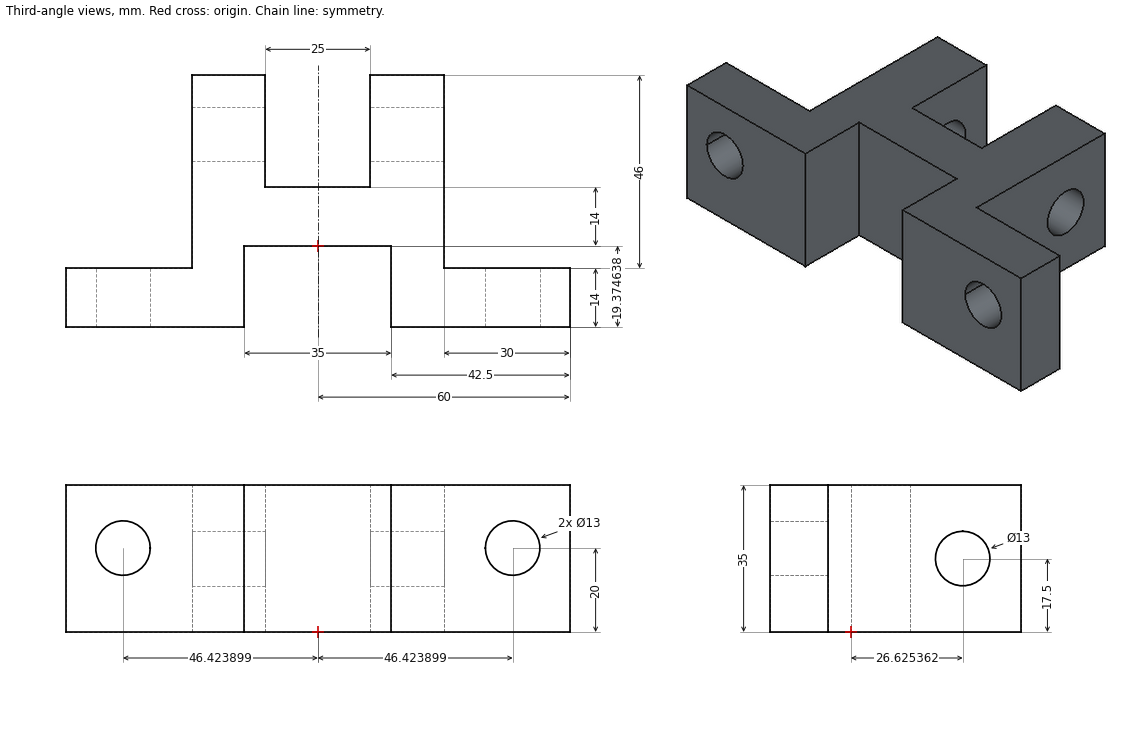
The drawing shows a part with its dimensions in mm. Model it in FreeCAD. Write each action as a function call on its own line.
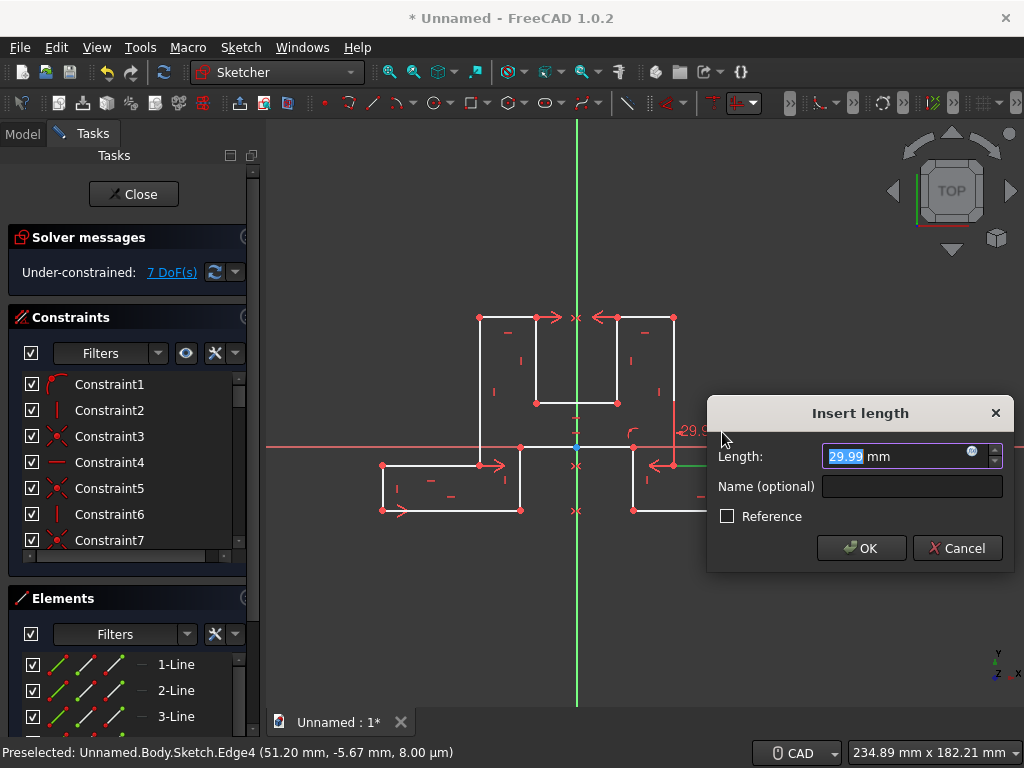
text(30)
key(Return)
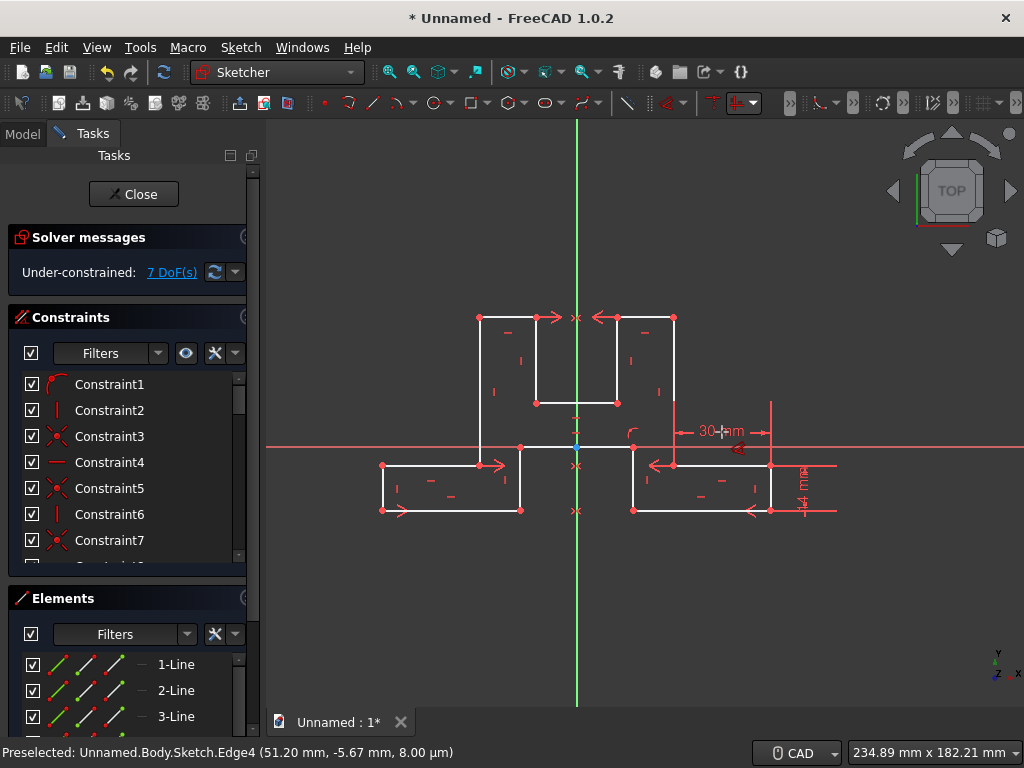
click(674, 421)
click(708, 392)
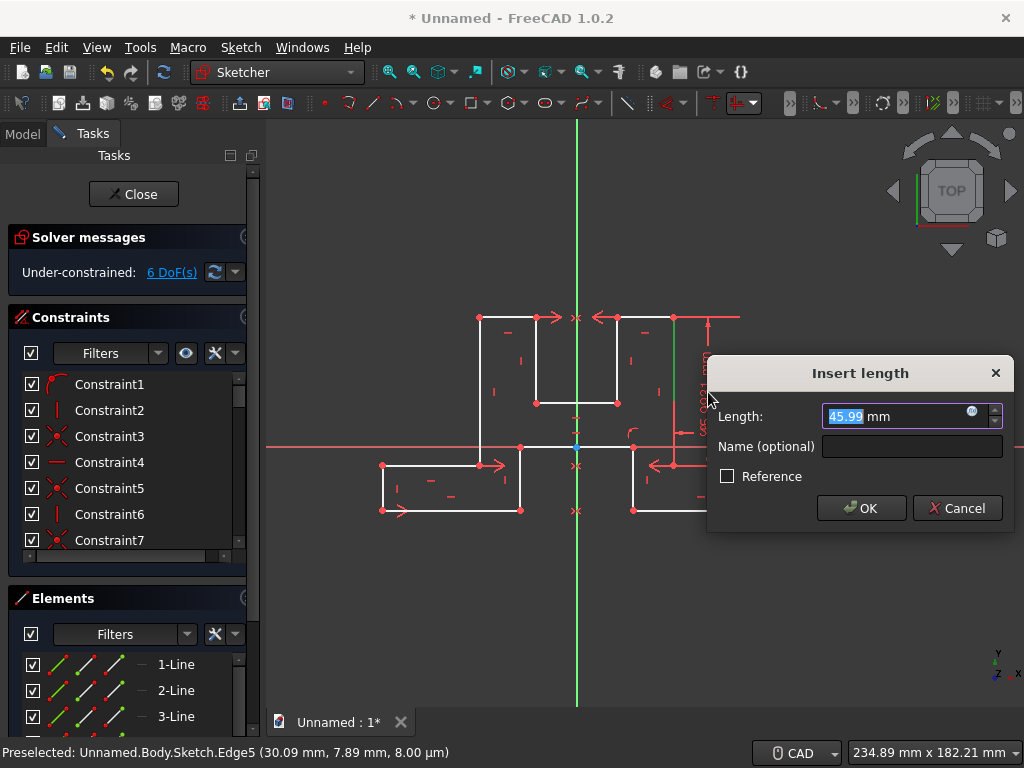
text(46)
key(Return)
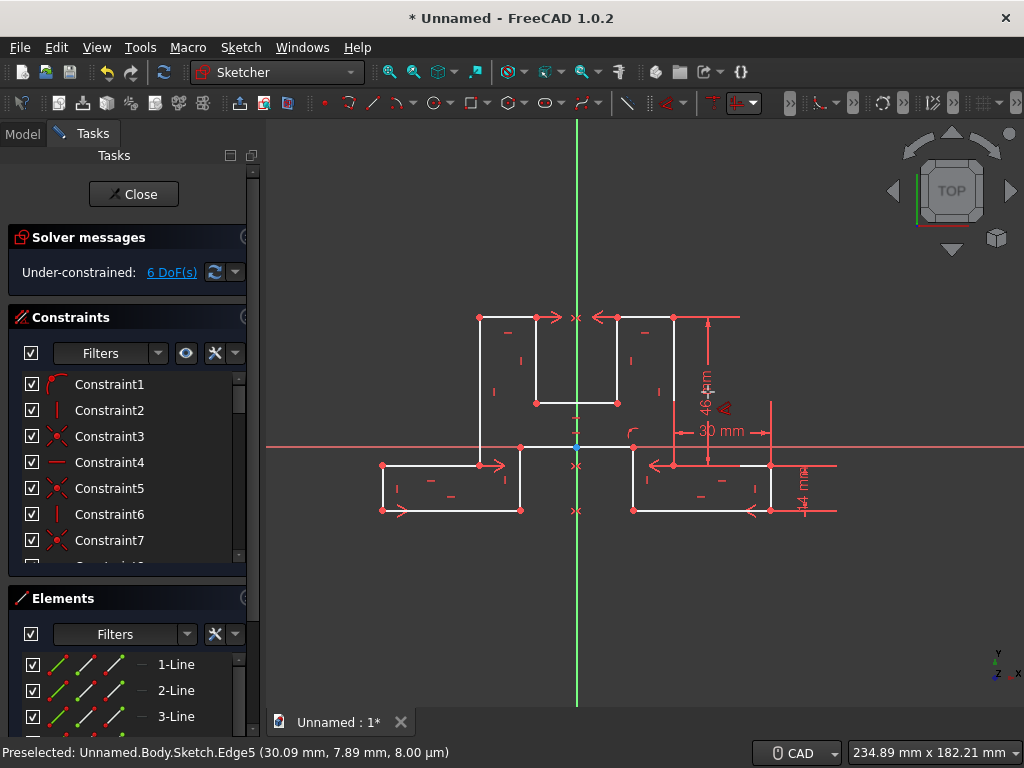
click(593, 403)
click(558, 369)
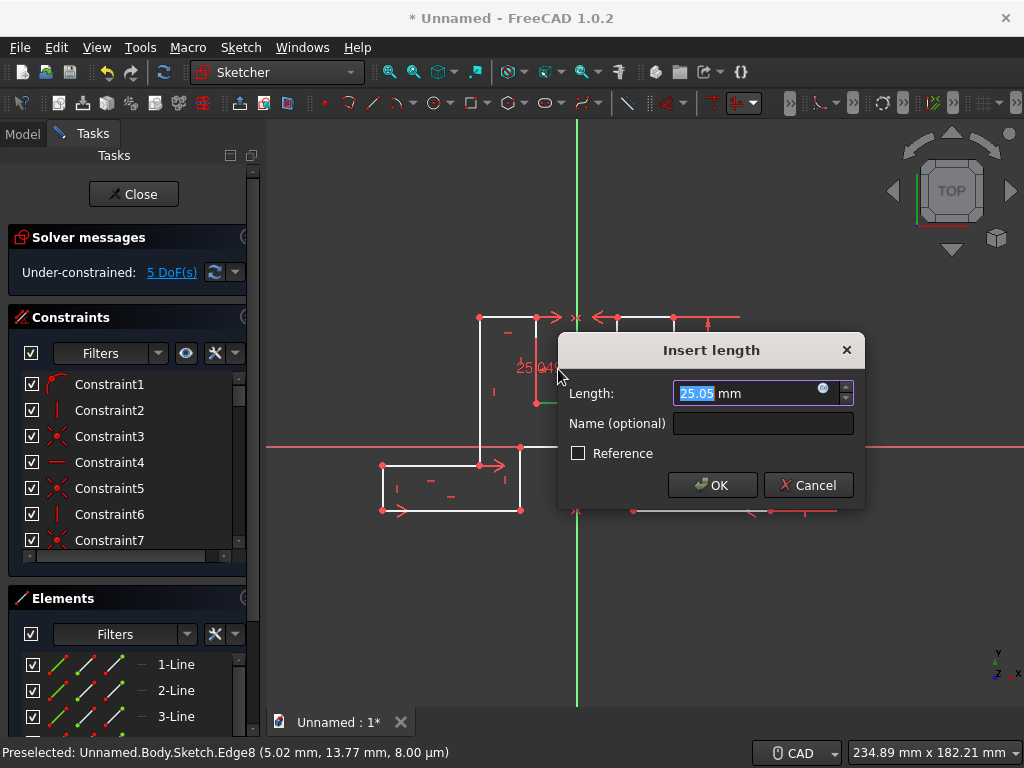
text(25)
key(Return)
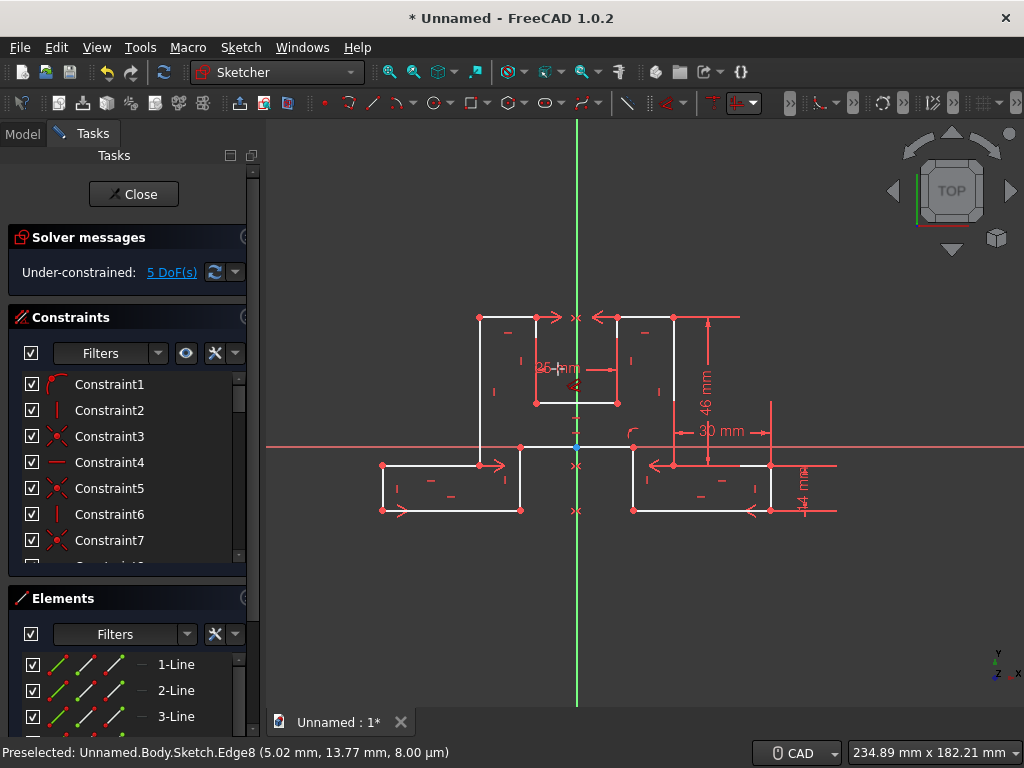
click(554, 447)
click(551, 481)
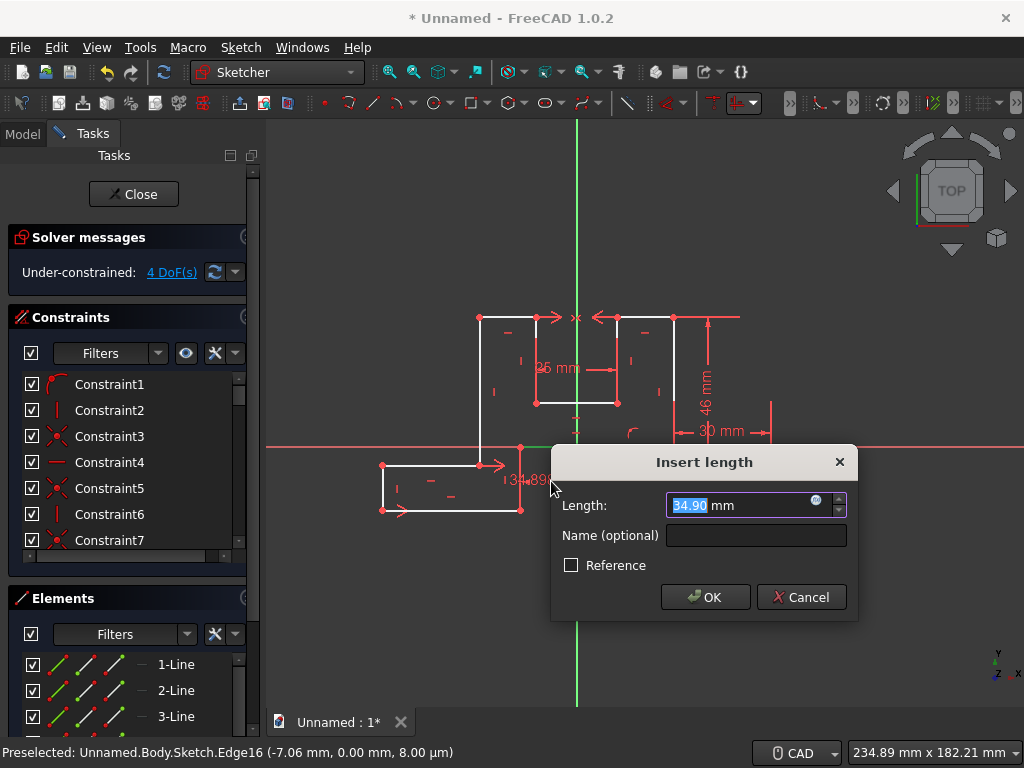
text(35)
key(Return)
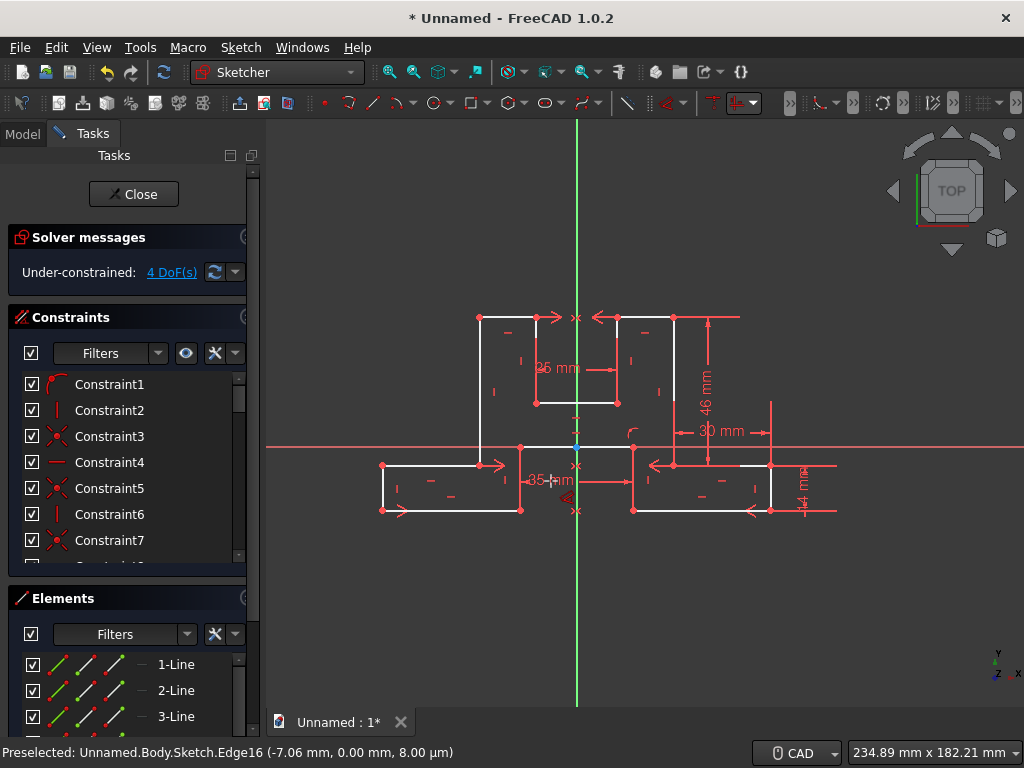
click(771, 511)
click(674, 545)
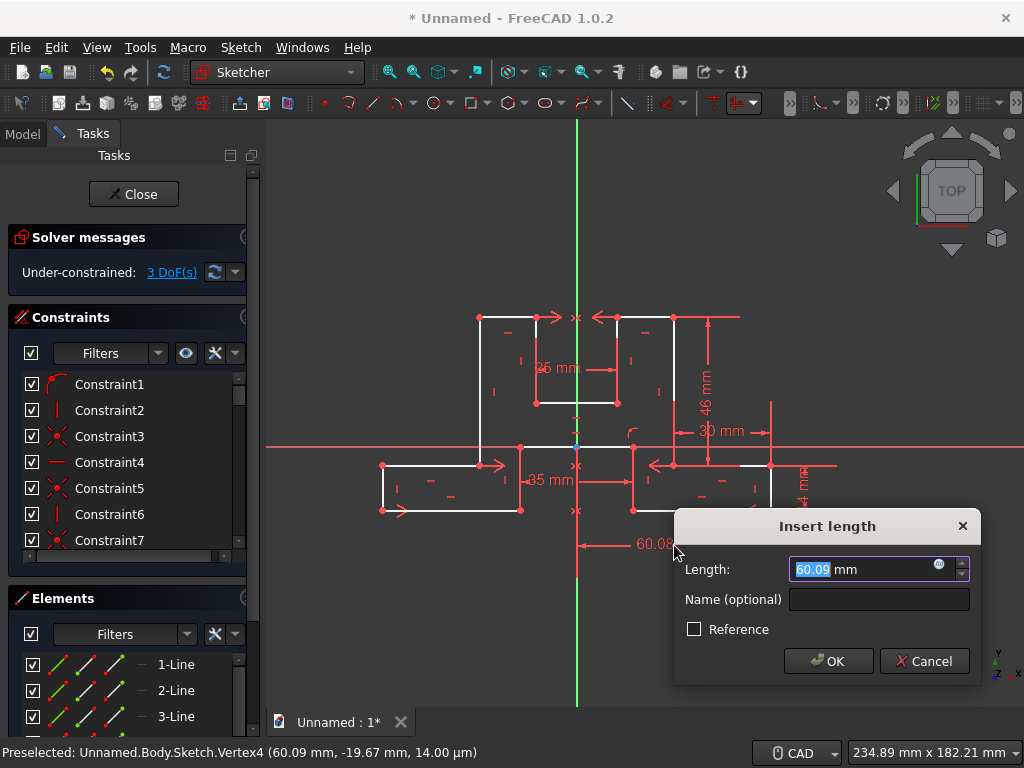
text(60)
key(Return)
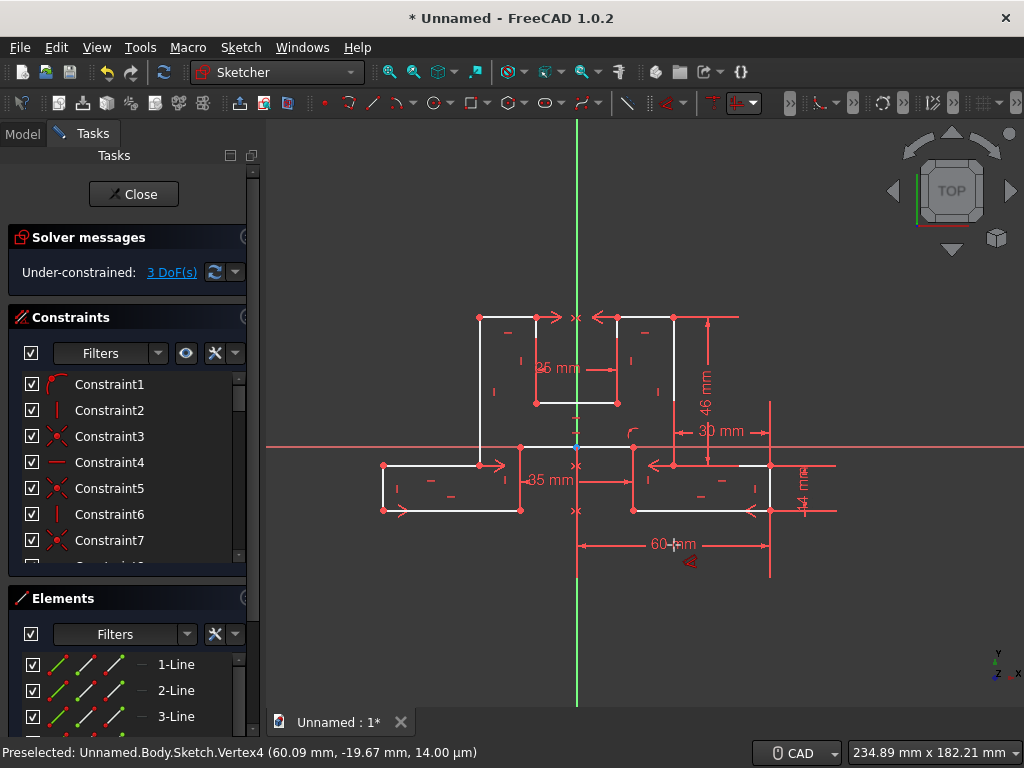
click(617, 403)
click(651, 425)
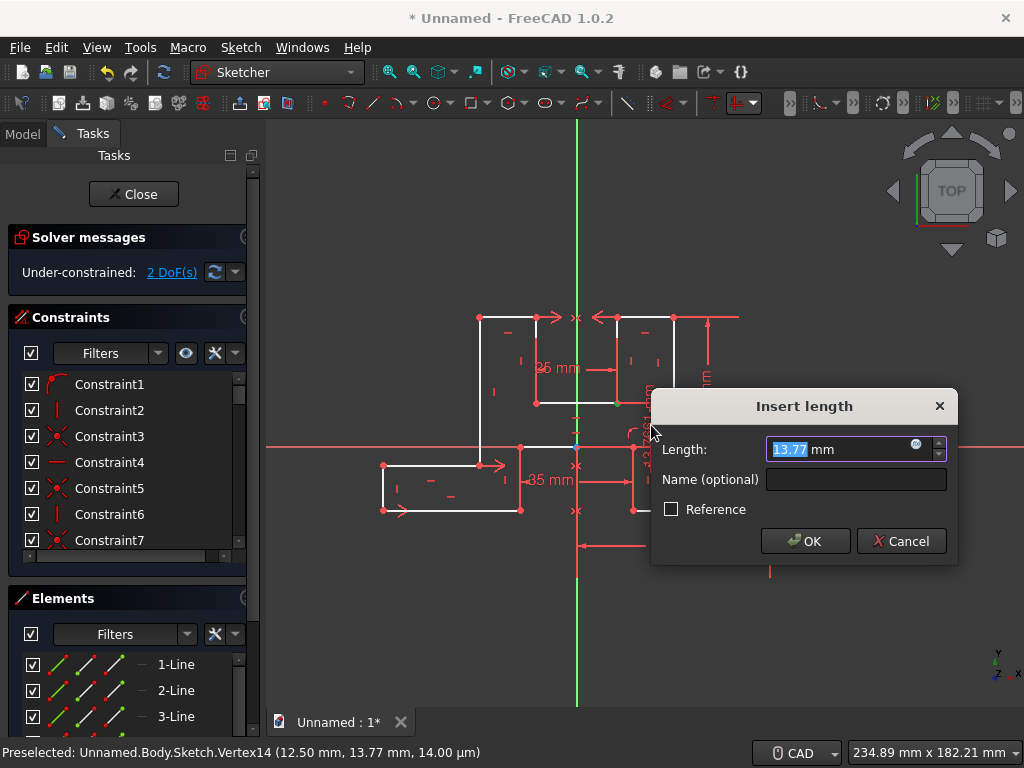
text(14)
key(Return)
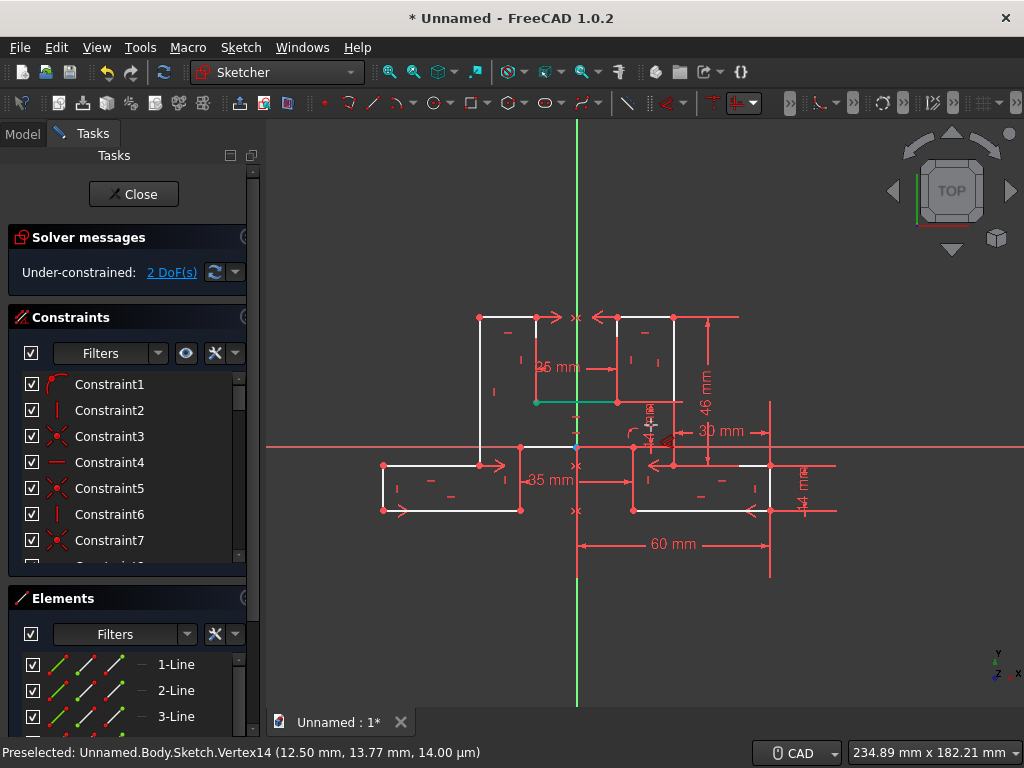
click(674, 511)
click(750, 545)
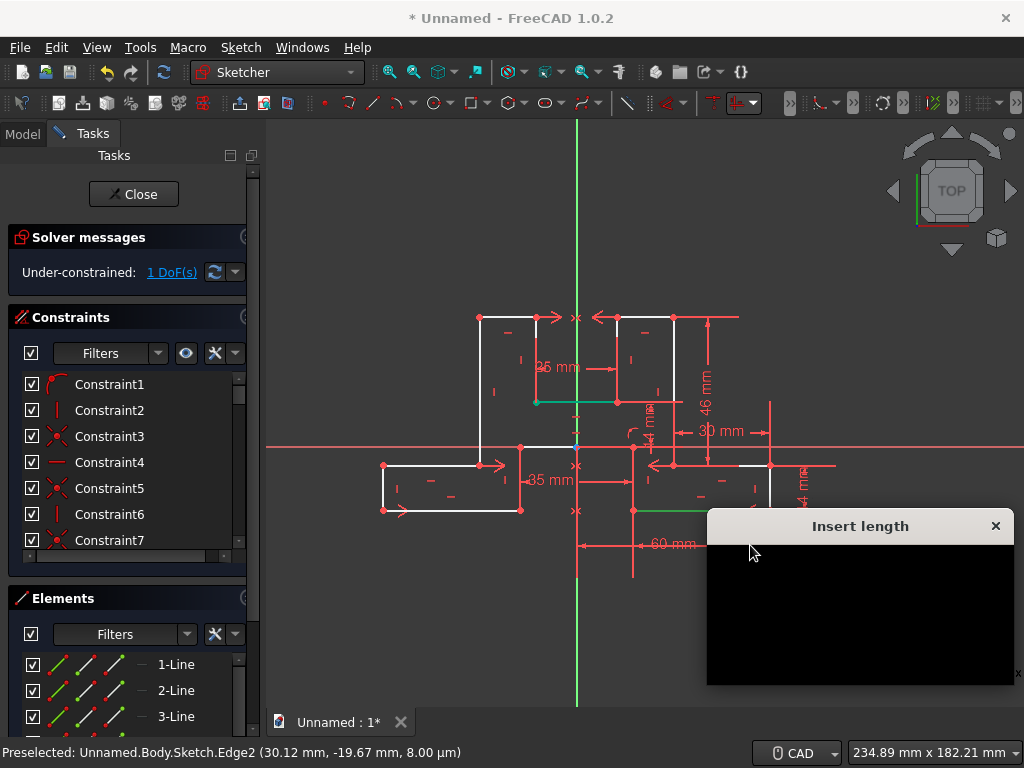
text(42.5)
key(Return)